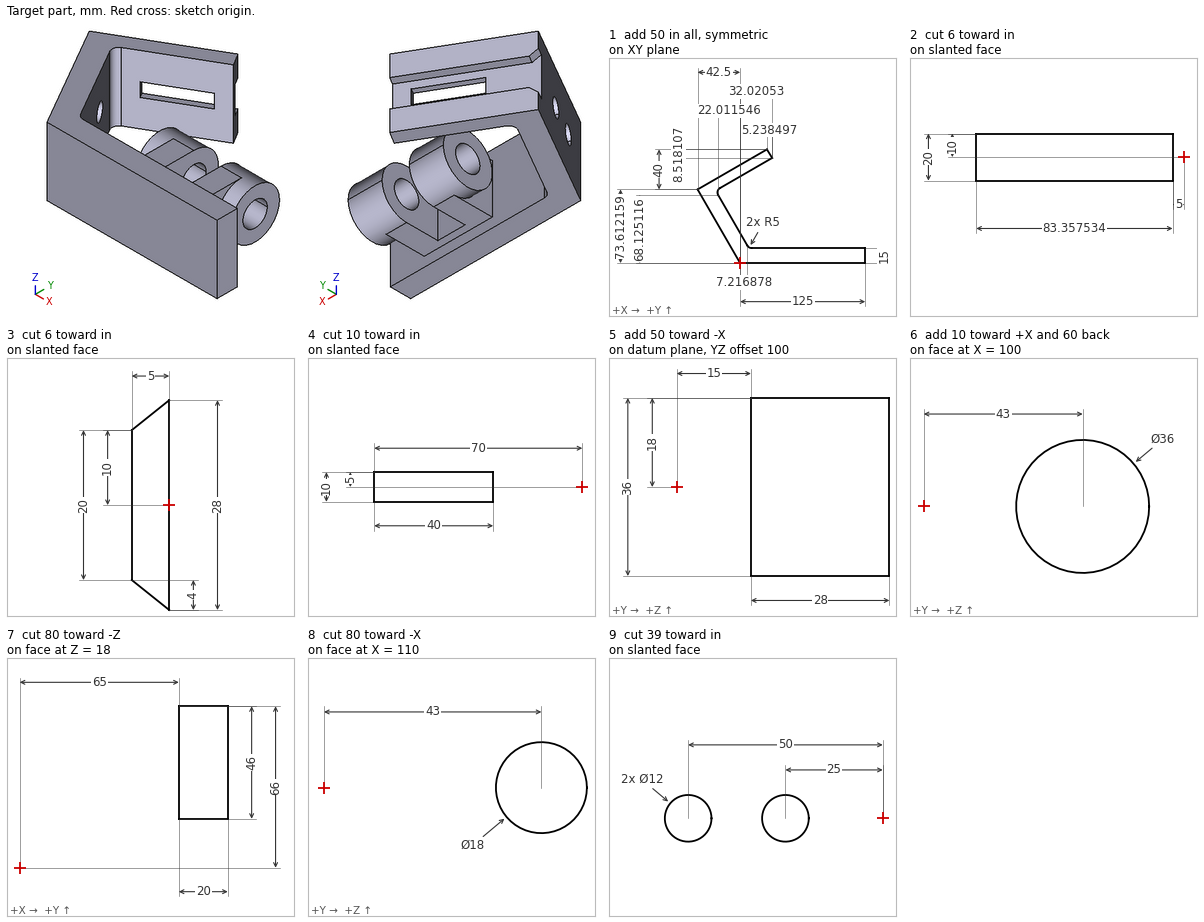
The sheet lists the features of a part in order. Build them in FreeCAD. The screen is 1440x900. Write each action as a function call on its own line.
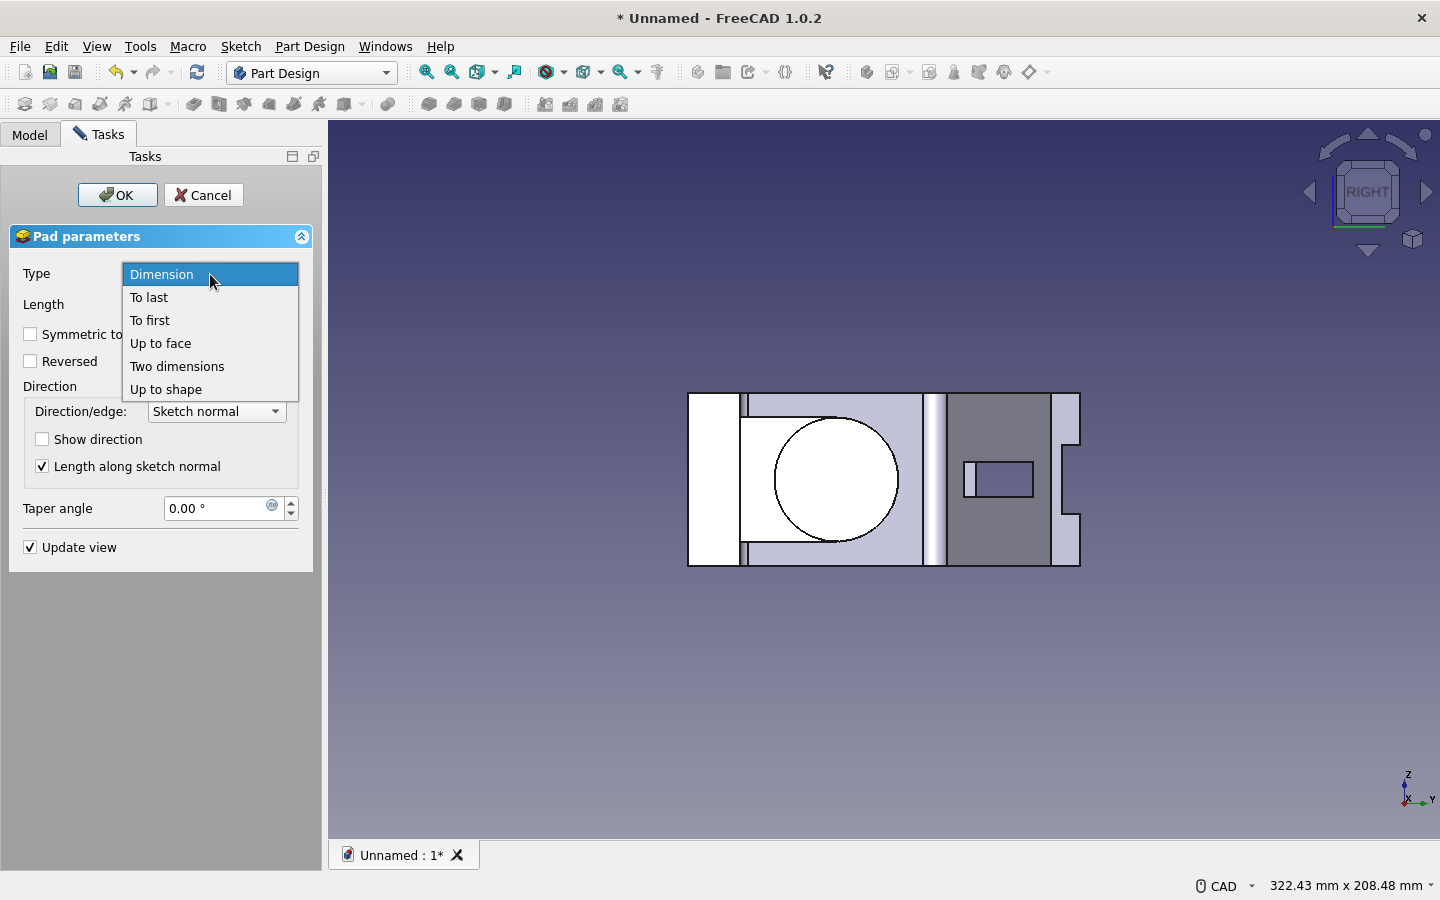
click(208, 366)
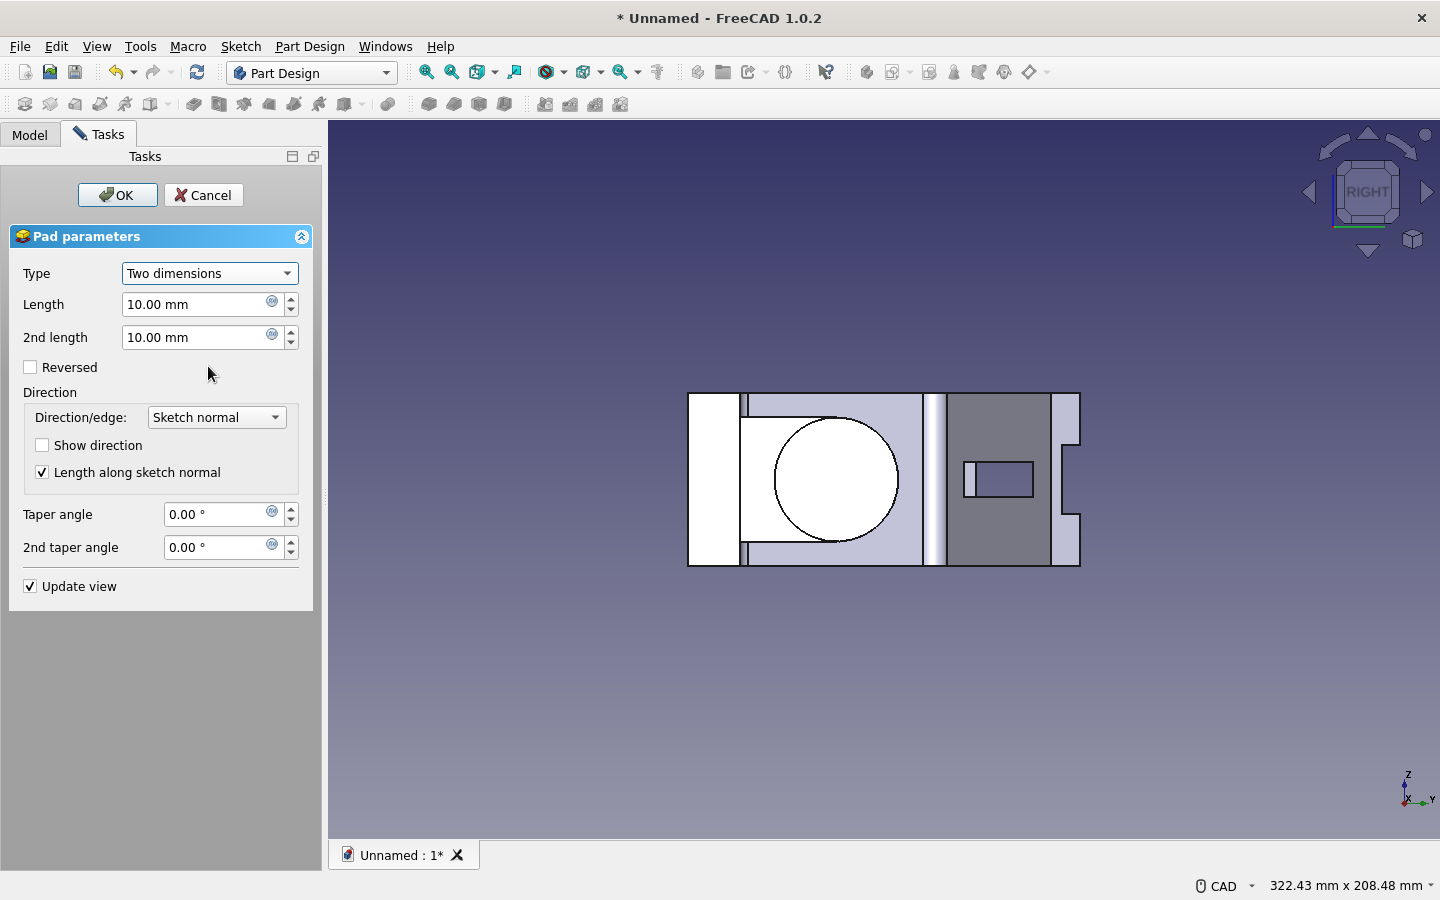
triple_click(204, 304)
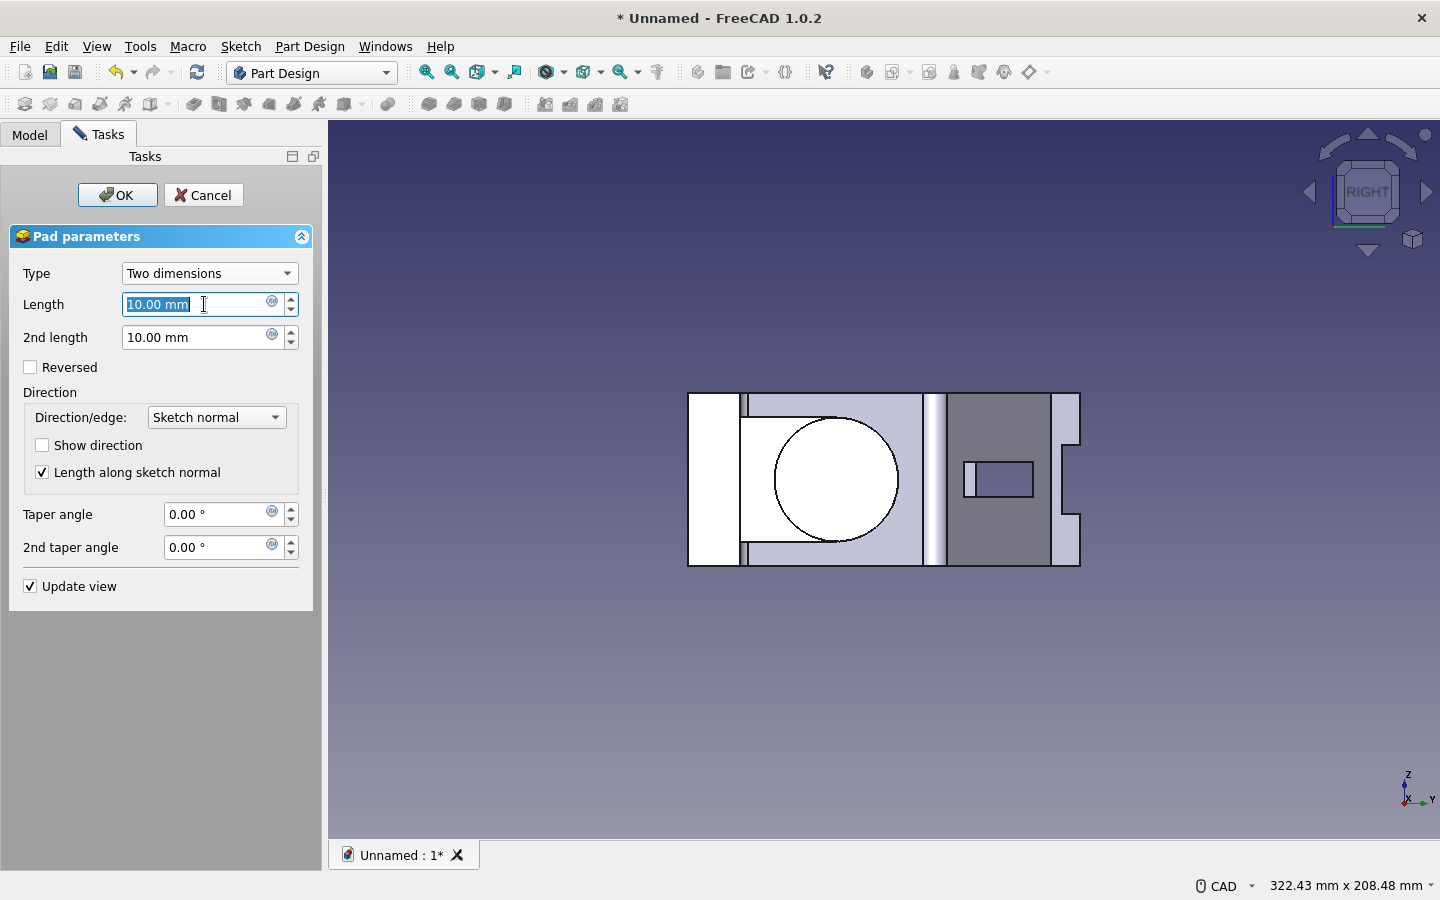
text(10)
key(Tab)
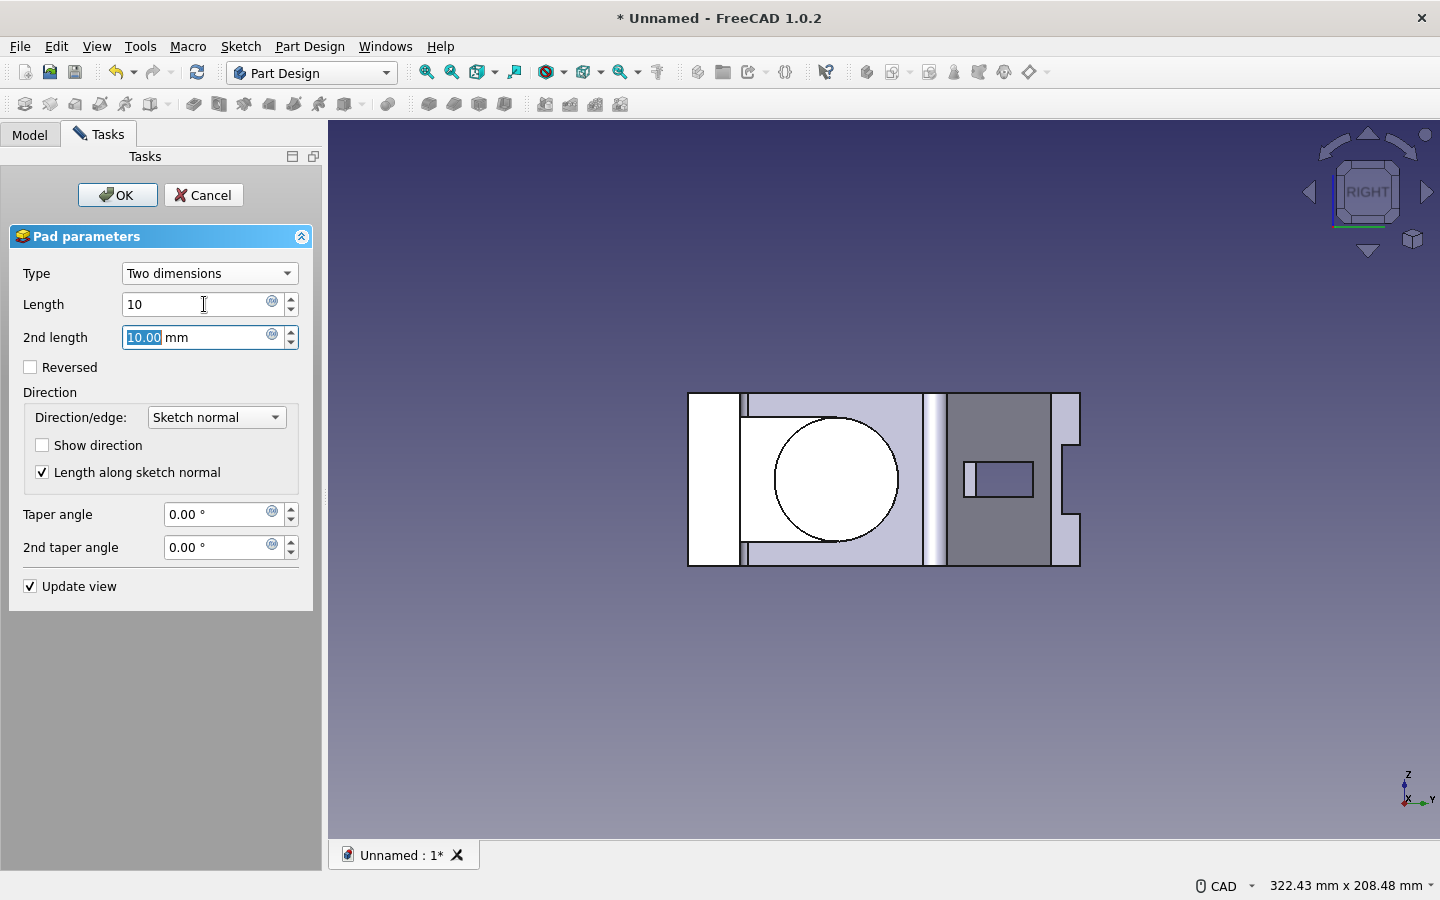
text(60)
key(Tab)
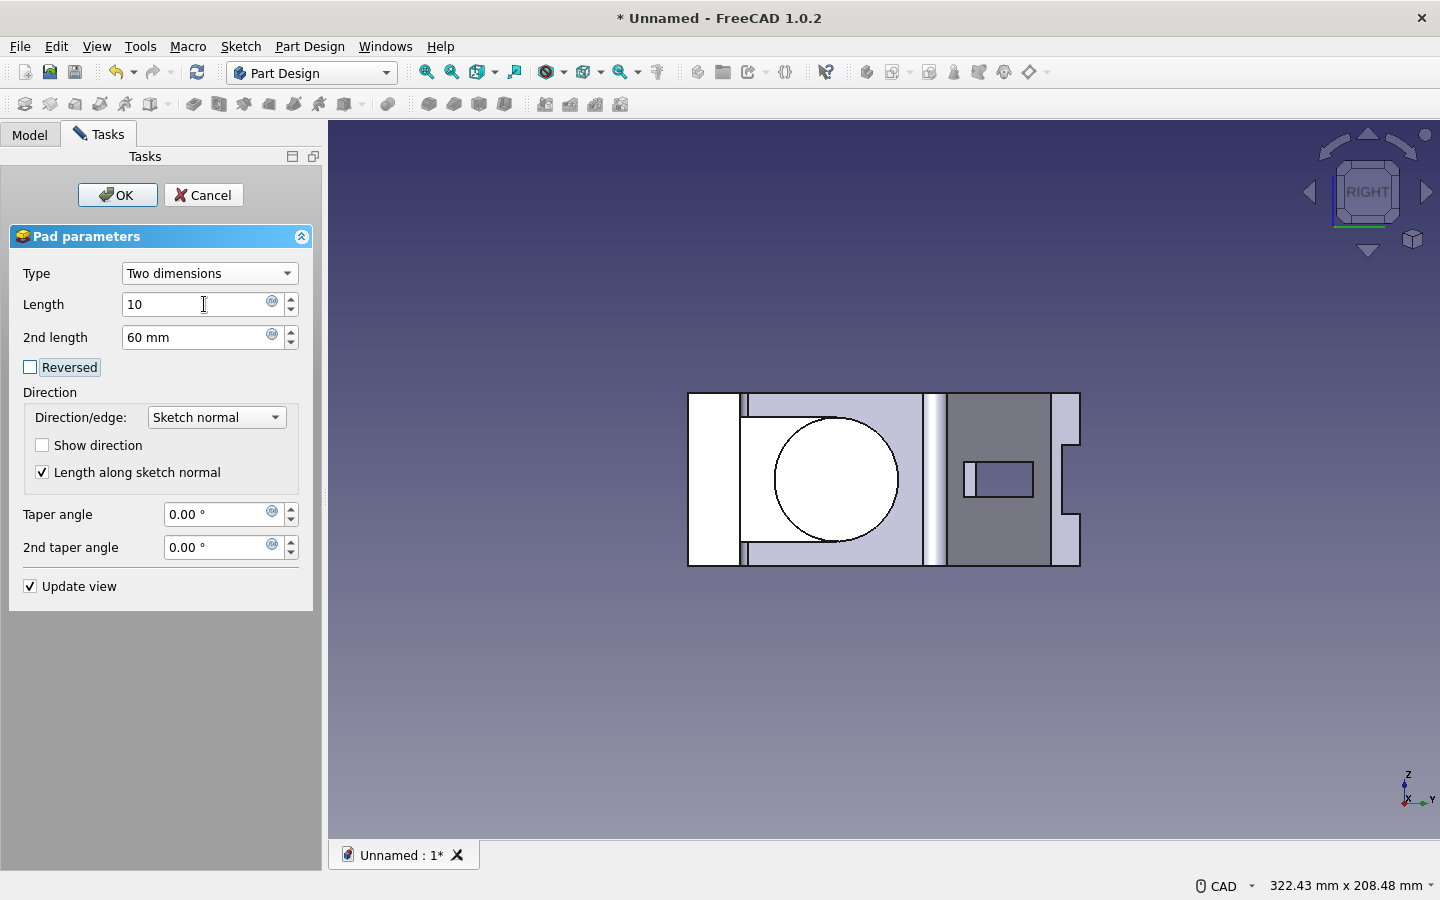
click(118, 195)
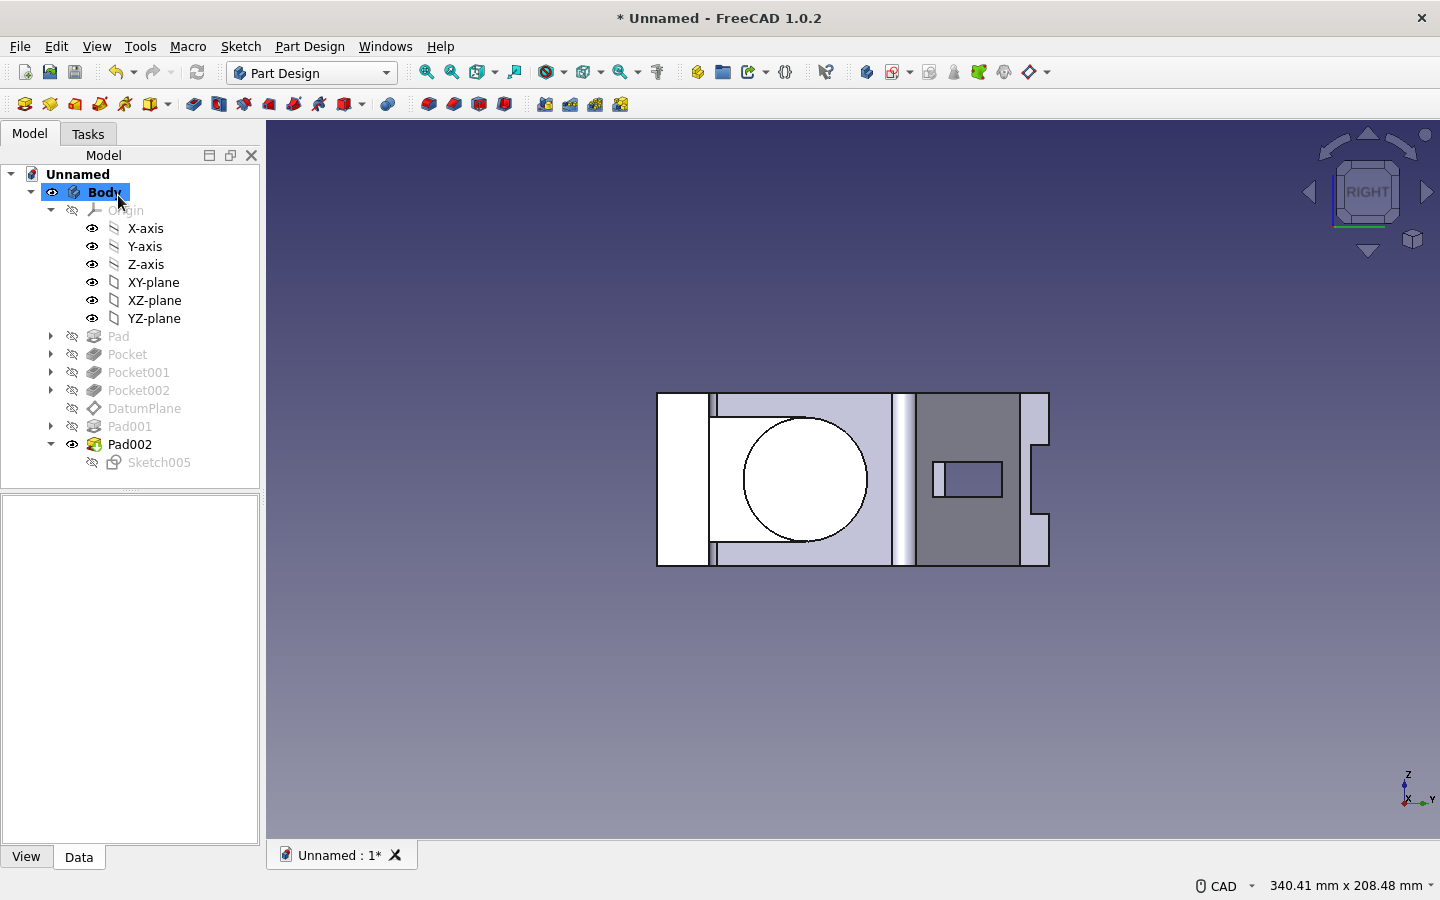
key(v)
key(f)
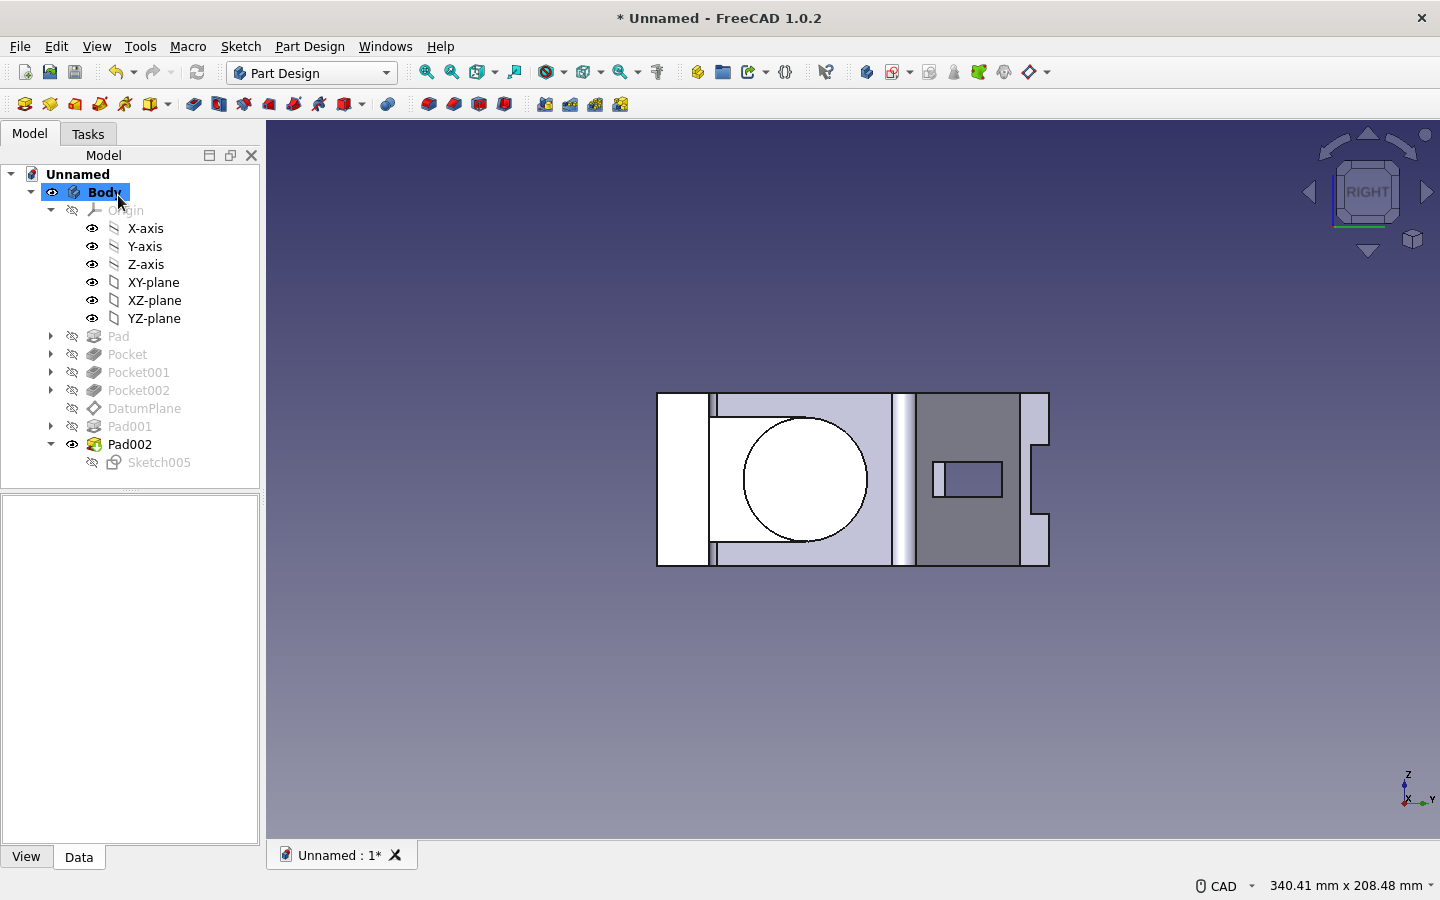
key(0)